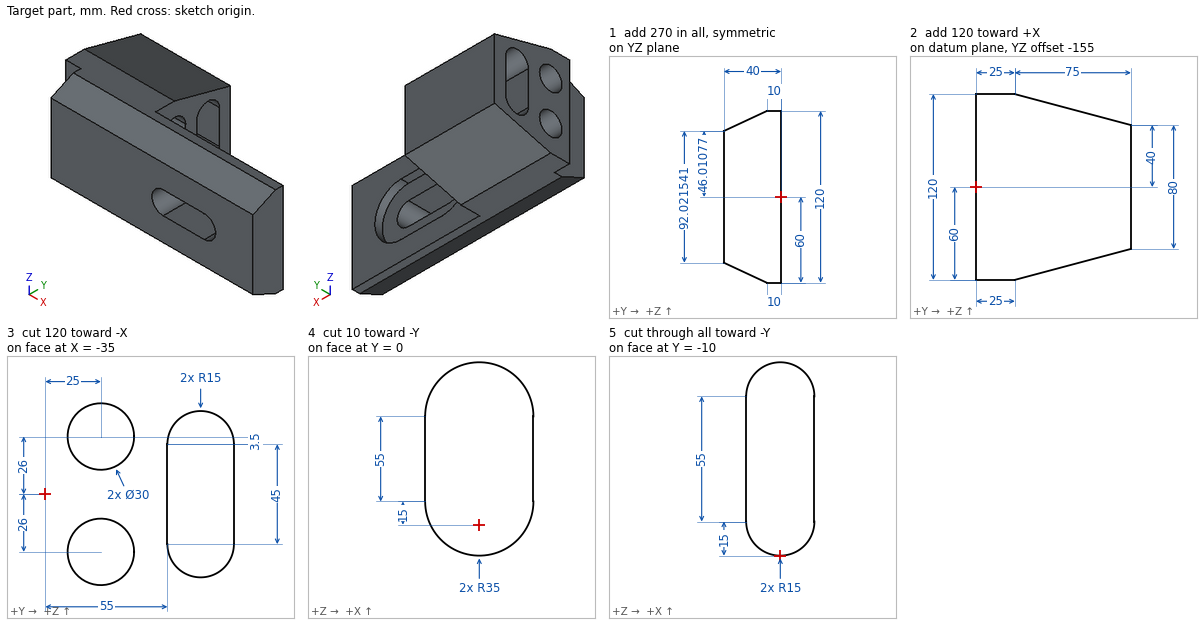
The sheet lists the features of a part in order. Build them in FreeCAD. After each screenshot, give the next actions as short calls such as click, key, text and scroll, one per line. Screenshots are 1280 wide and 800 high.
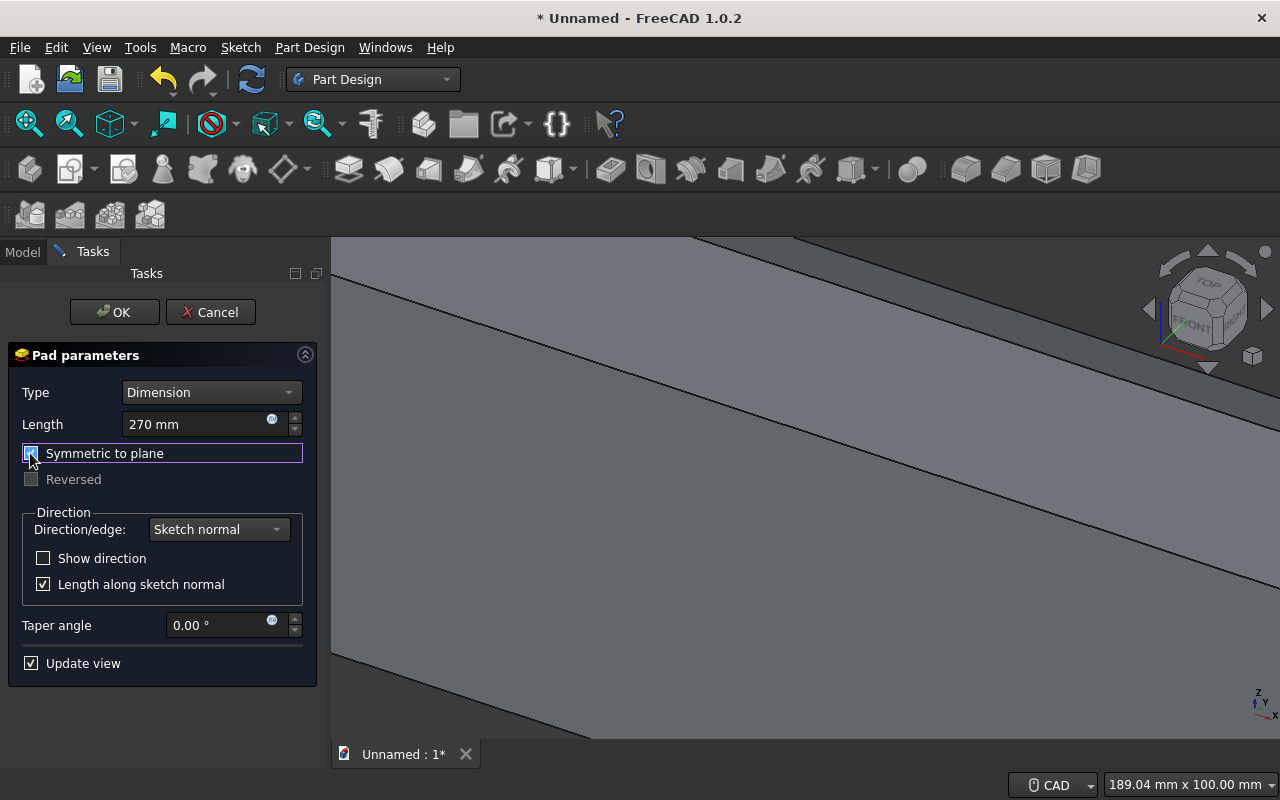
click(115, 312)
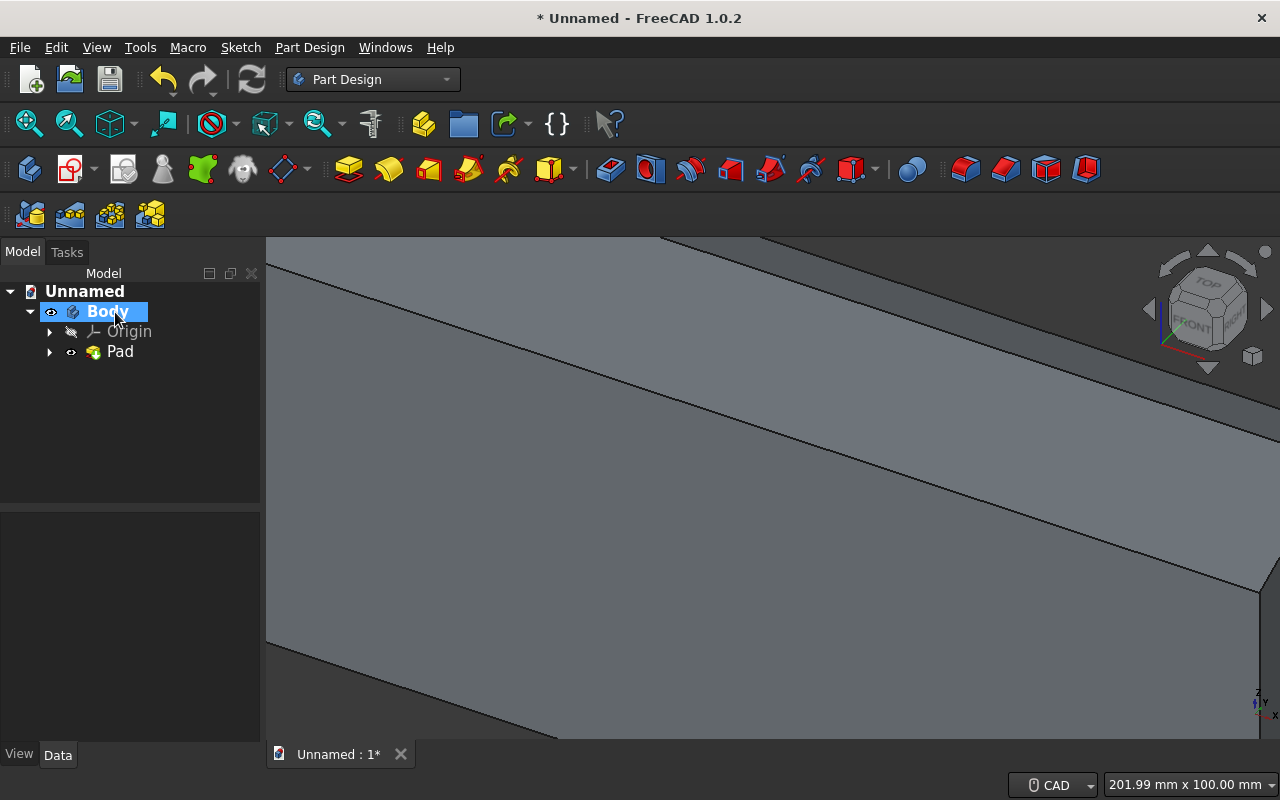
click(30, 124)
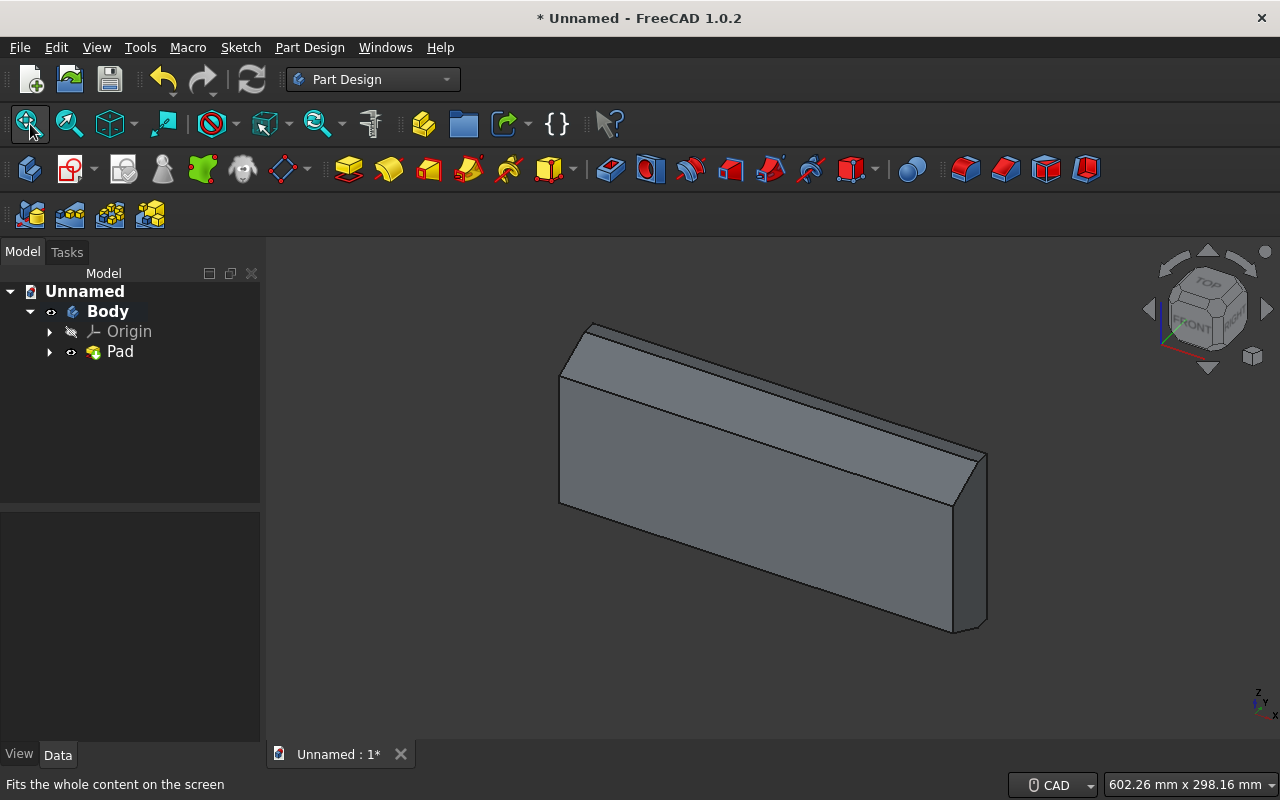
click(50, 332)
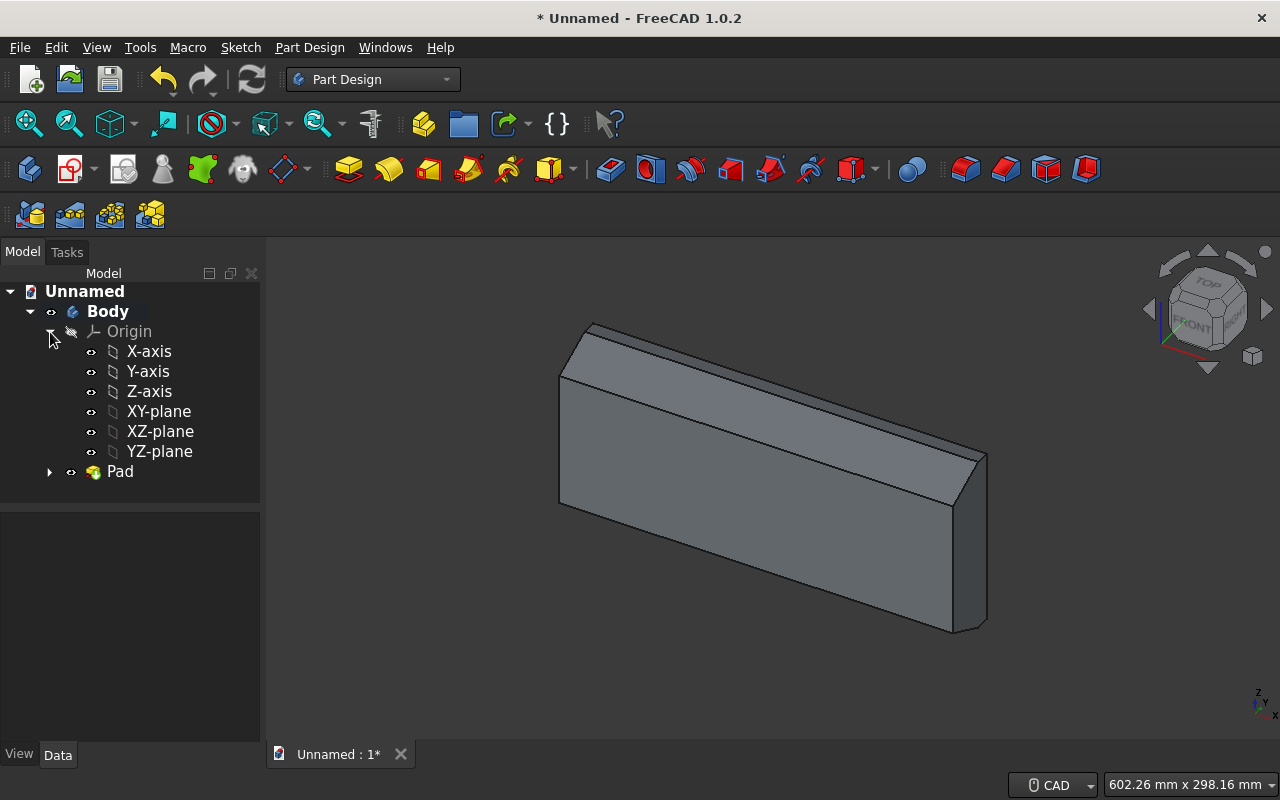
click(136, 452)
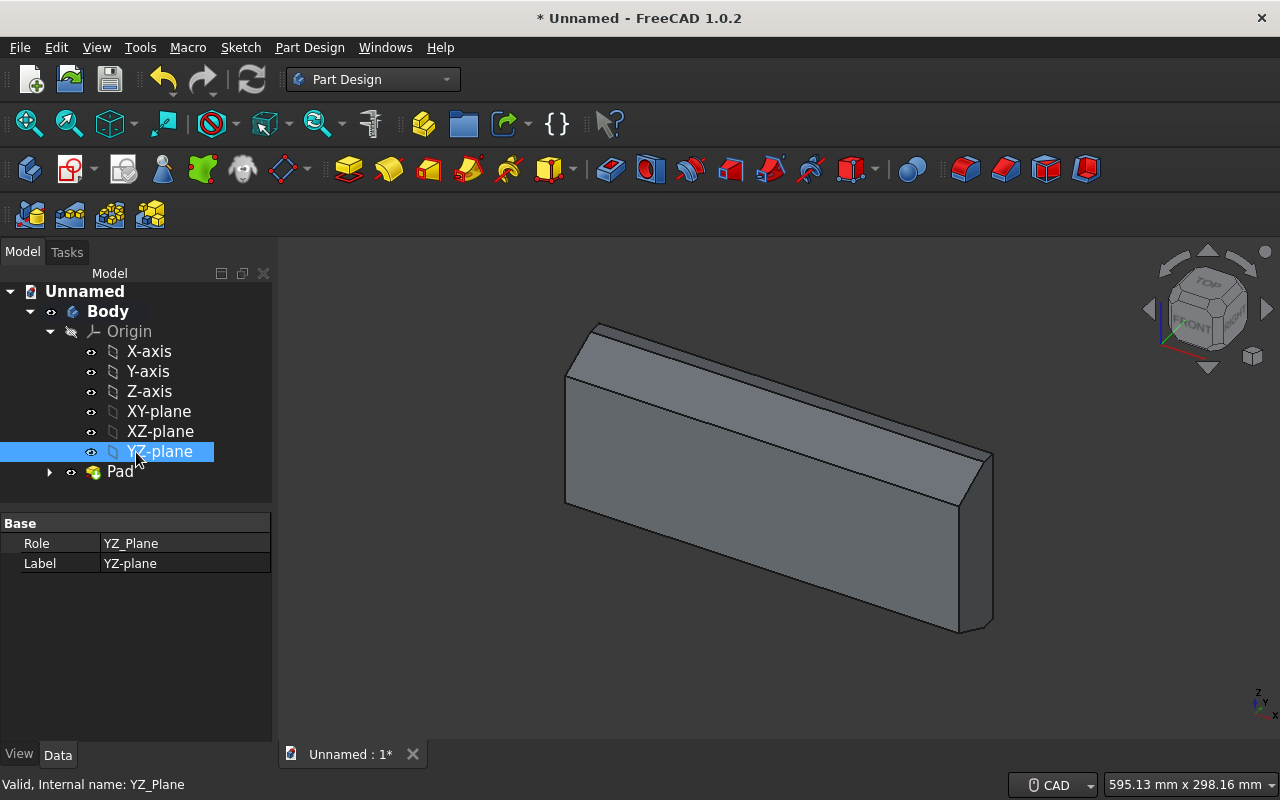
click(284, 170)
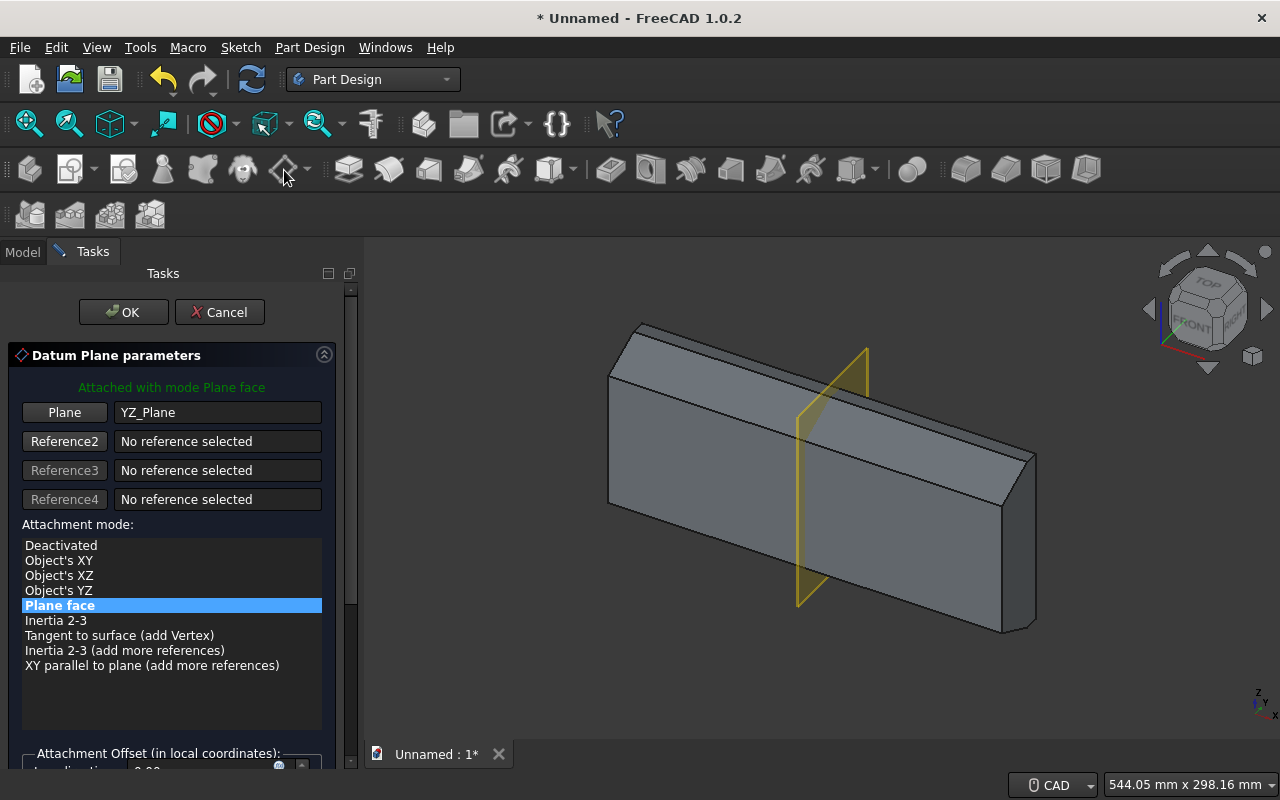
scroll(351, 526, down, 3)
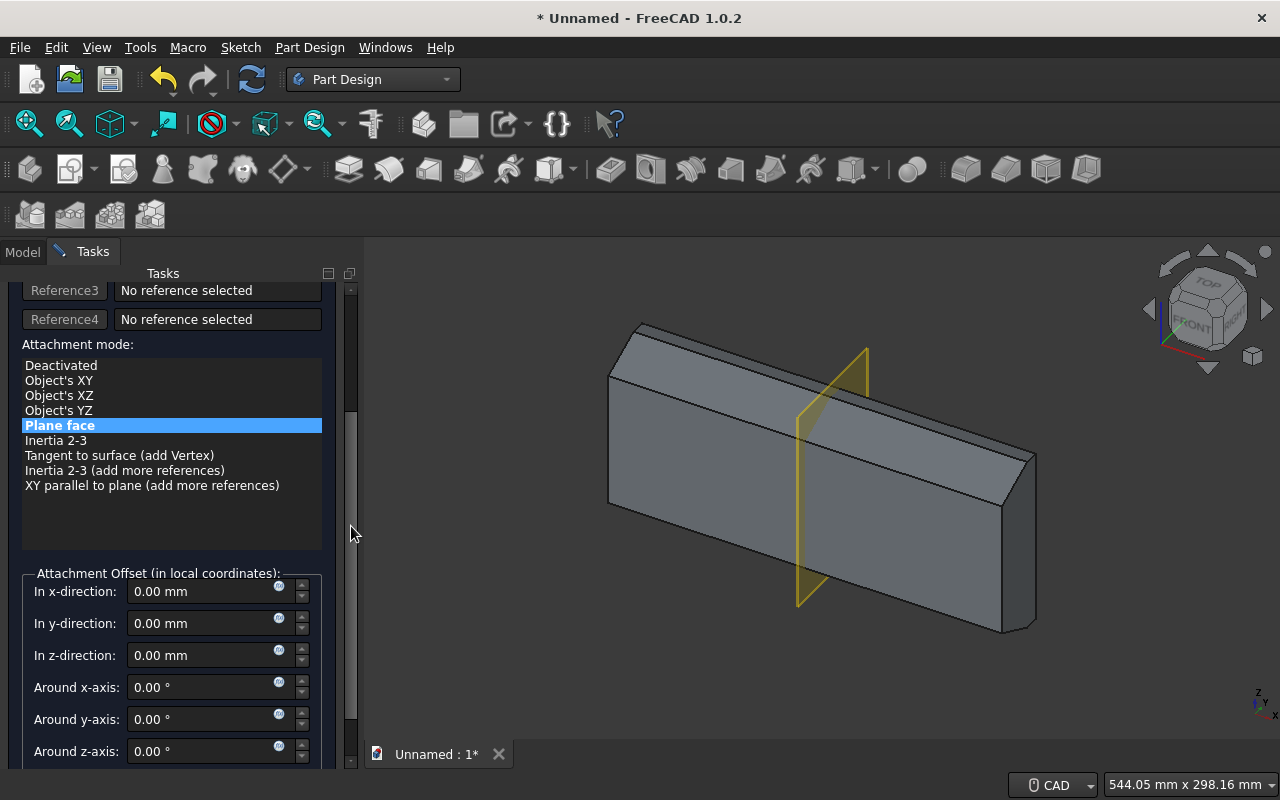
triple_click(210, 655)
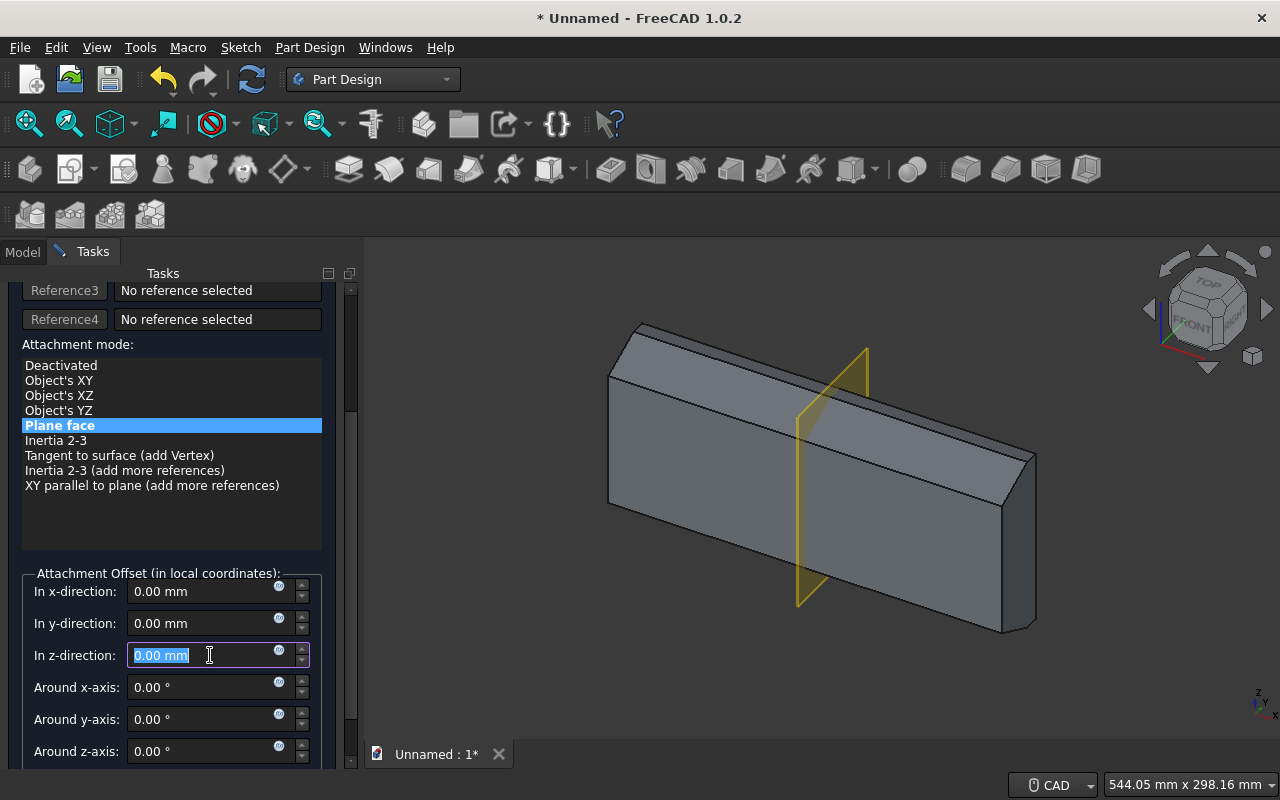
text(-155)
key(Tab)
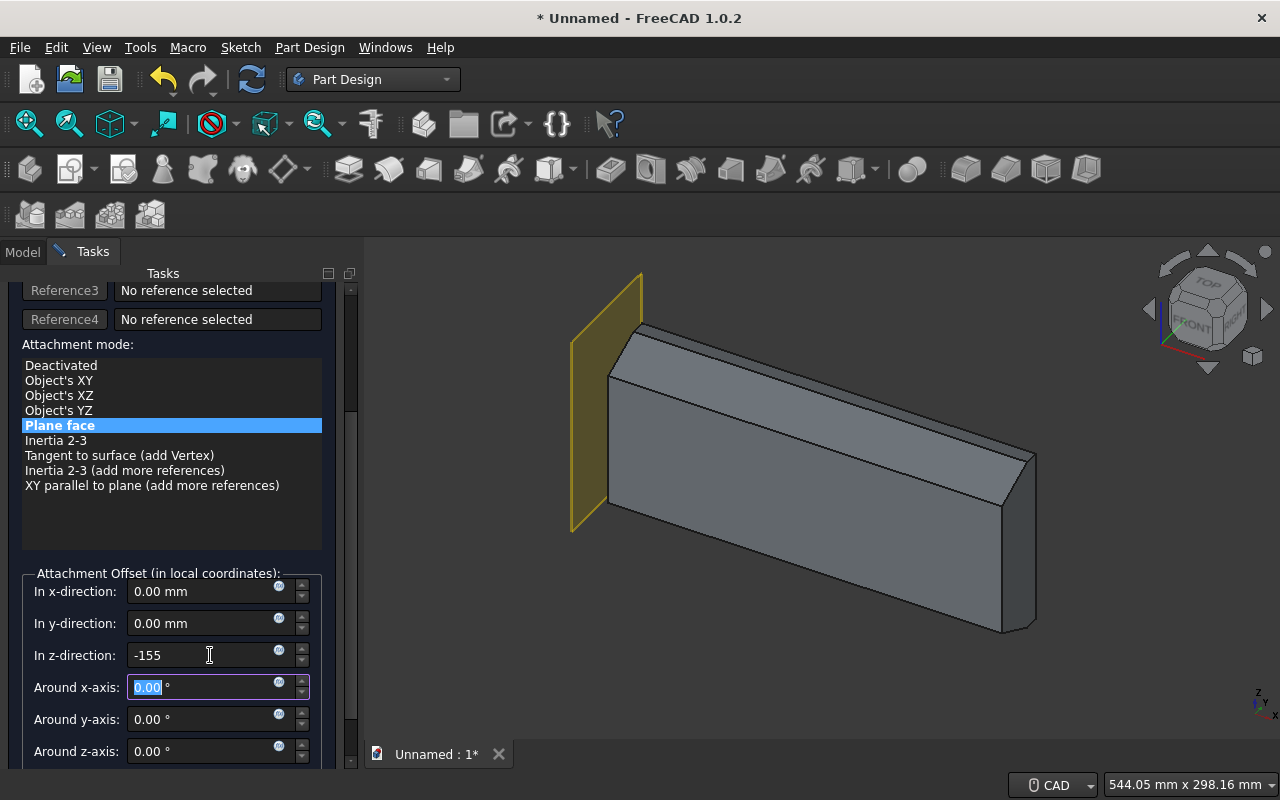
scroll(351, 526, up, 4)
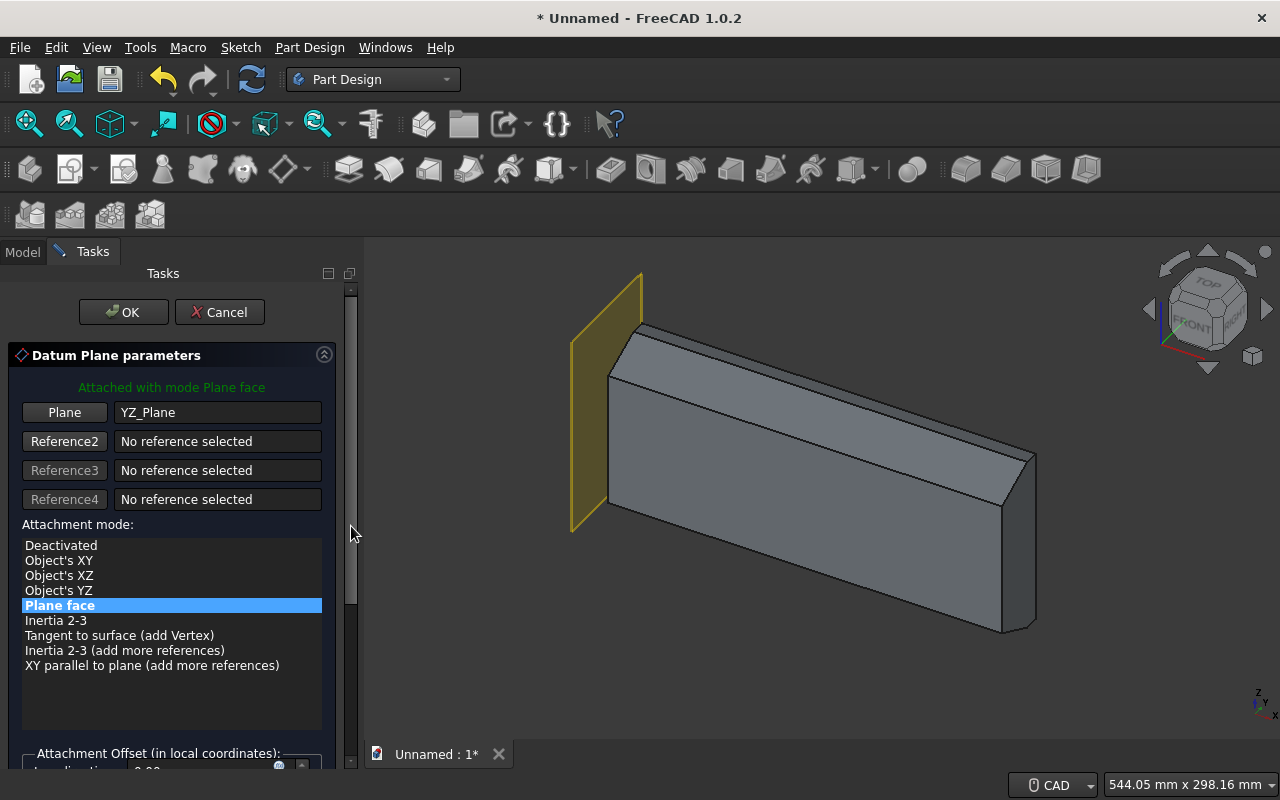
click(124, 312)